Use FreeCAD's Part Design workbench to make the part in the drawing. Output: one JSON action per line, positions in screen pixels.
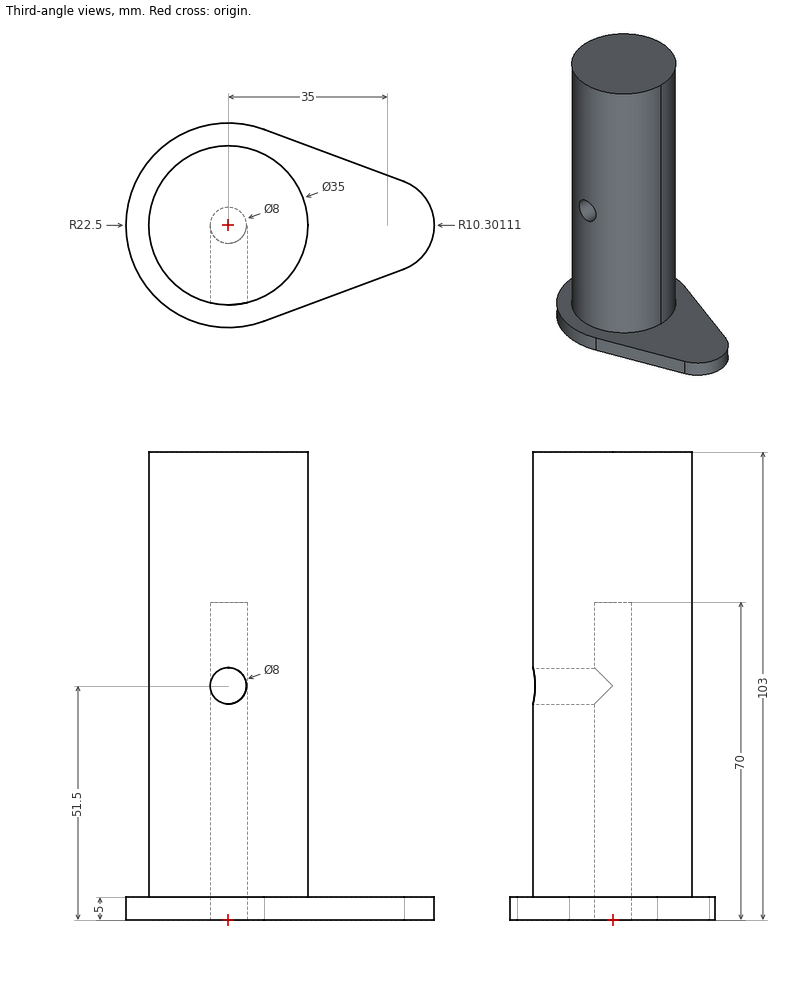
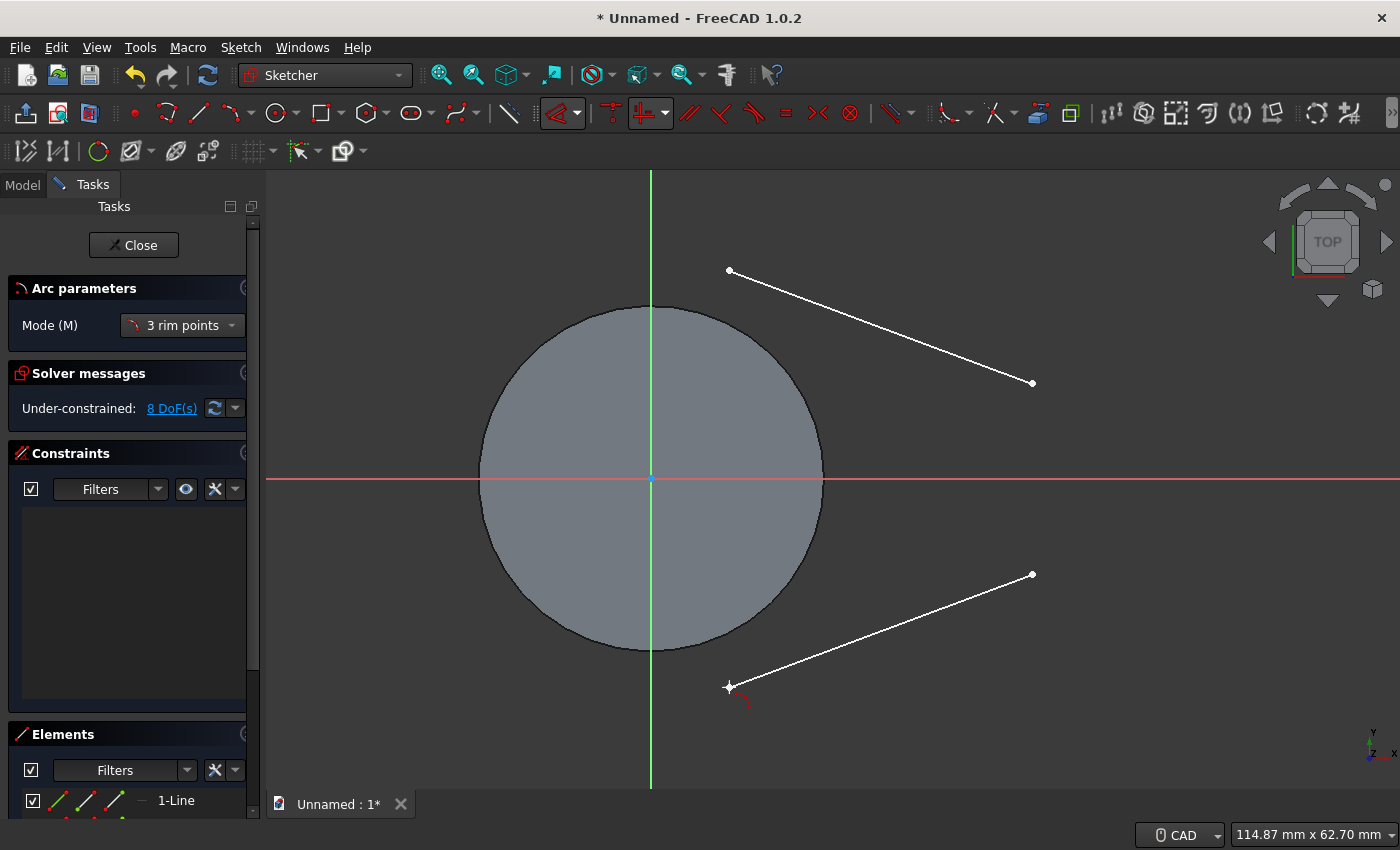
{"action": "left_click", "coordinate": [1032, 384]}
{"action": "left_click", "coordinate": [1032, 575]}
{"action": "left_click", "coordinate": [1096, 503]}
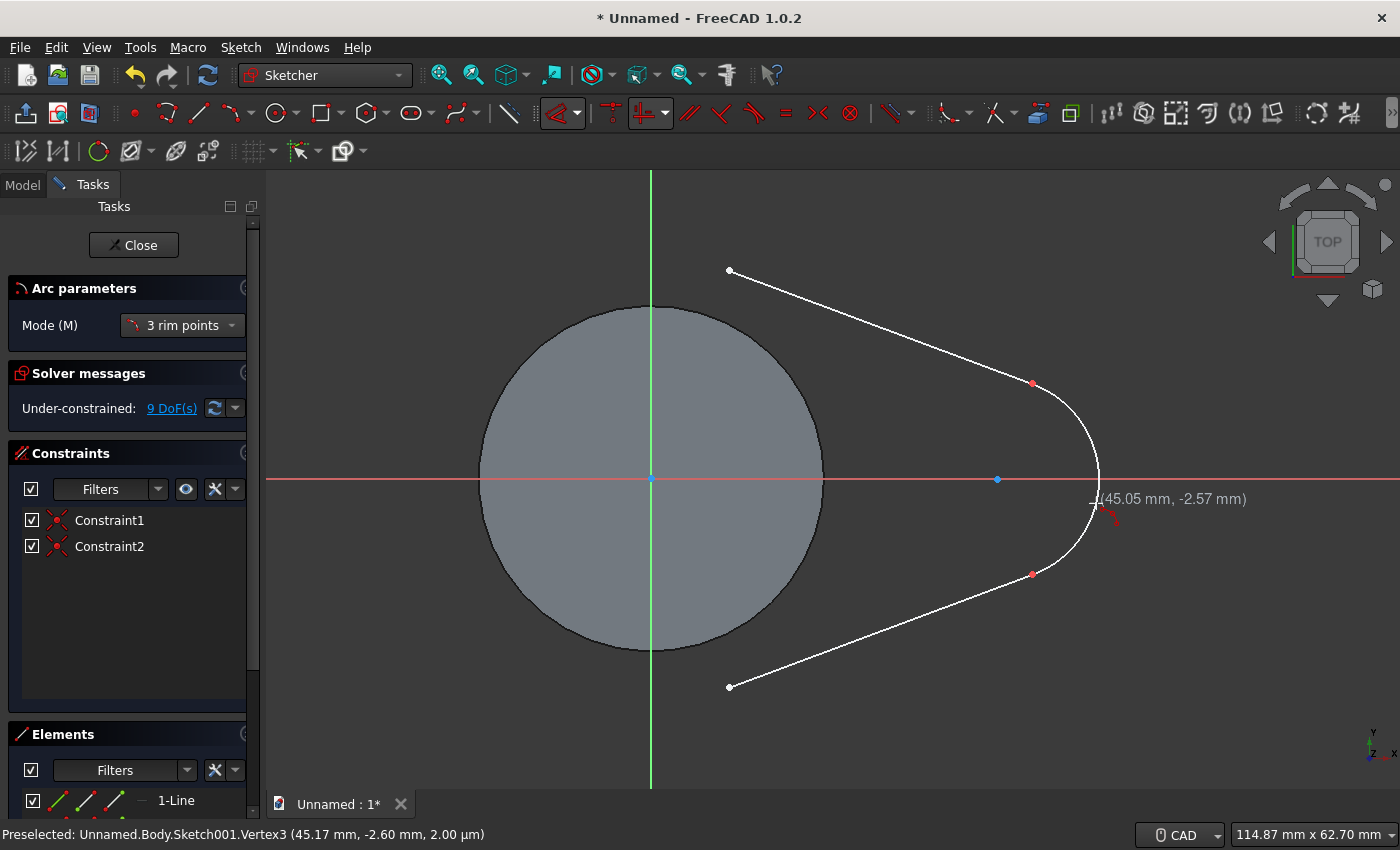
{"action": "left_click", "coordinate": [729, 688]}
{"action": "left_click", "coordinate": [729, 271]}
{"action": "left_click", "coordinate": [445, 395]}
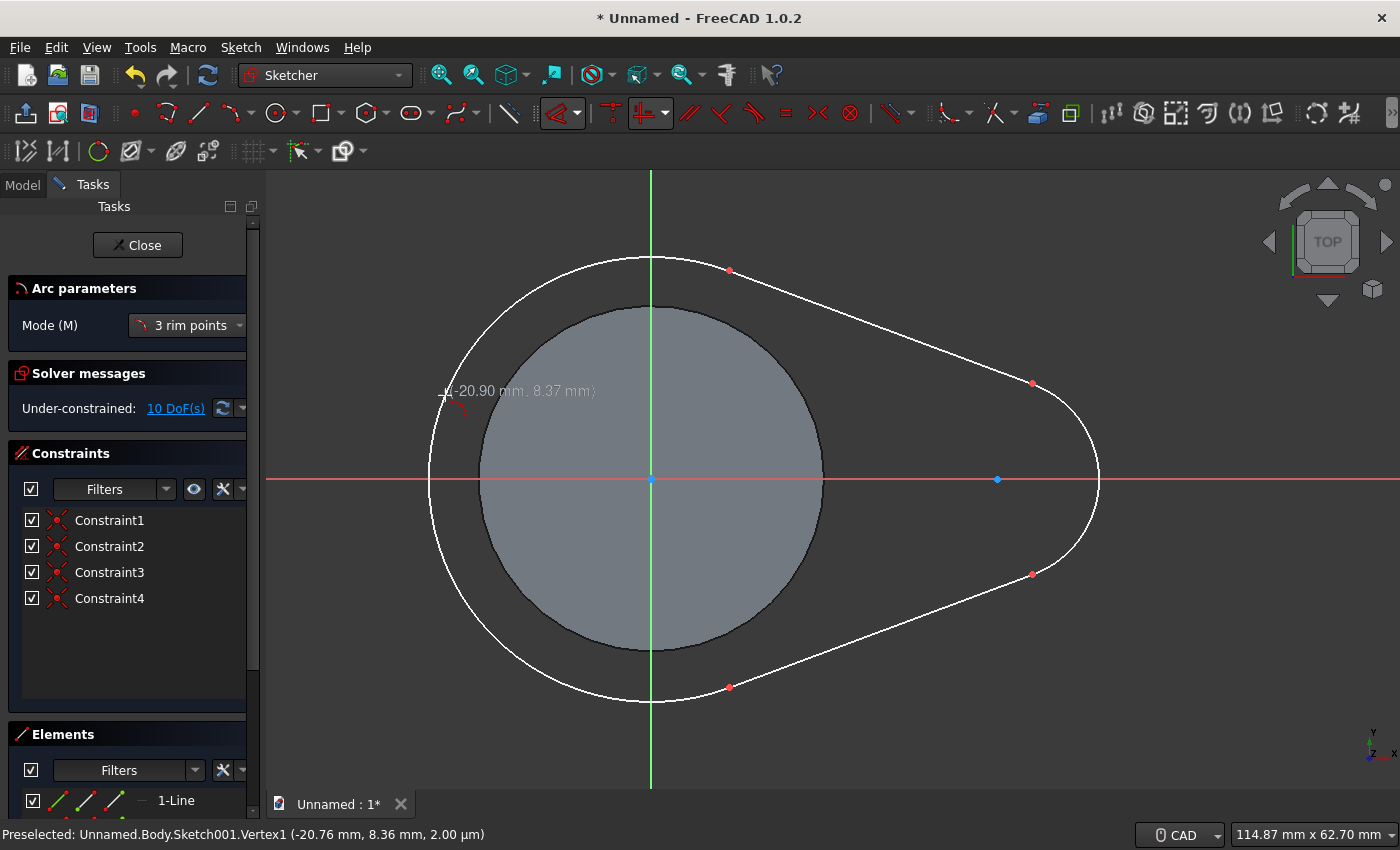
{"action": "left_click", "coordinate": [276, 114]}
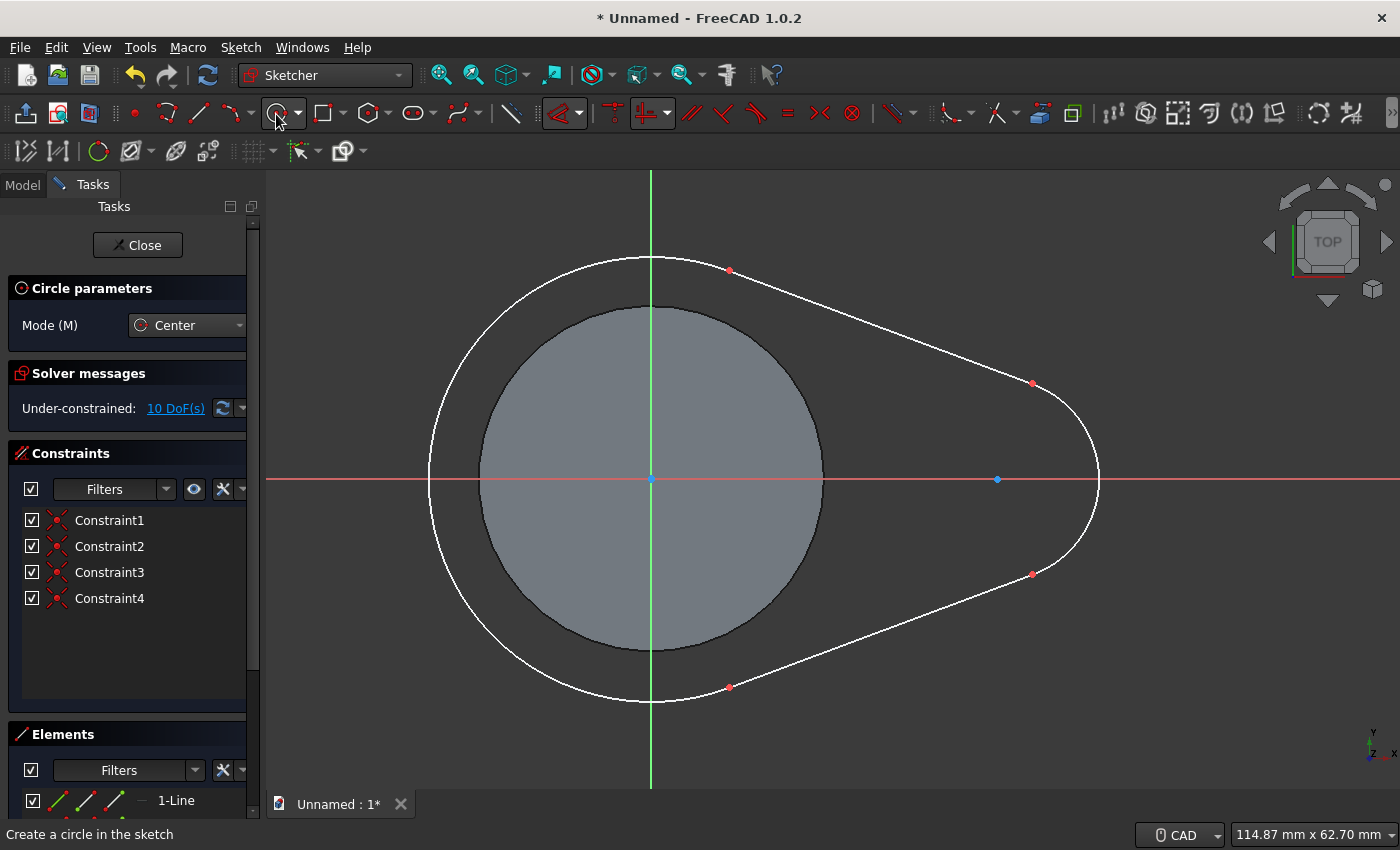
{"action": "left_click", "coordinate": [651, 479]}
{"action": "left_click", "coordinate": [773, 357]}
{"action": "key", "text": "Escape"}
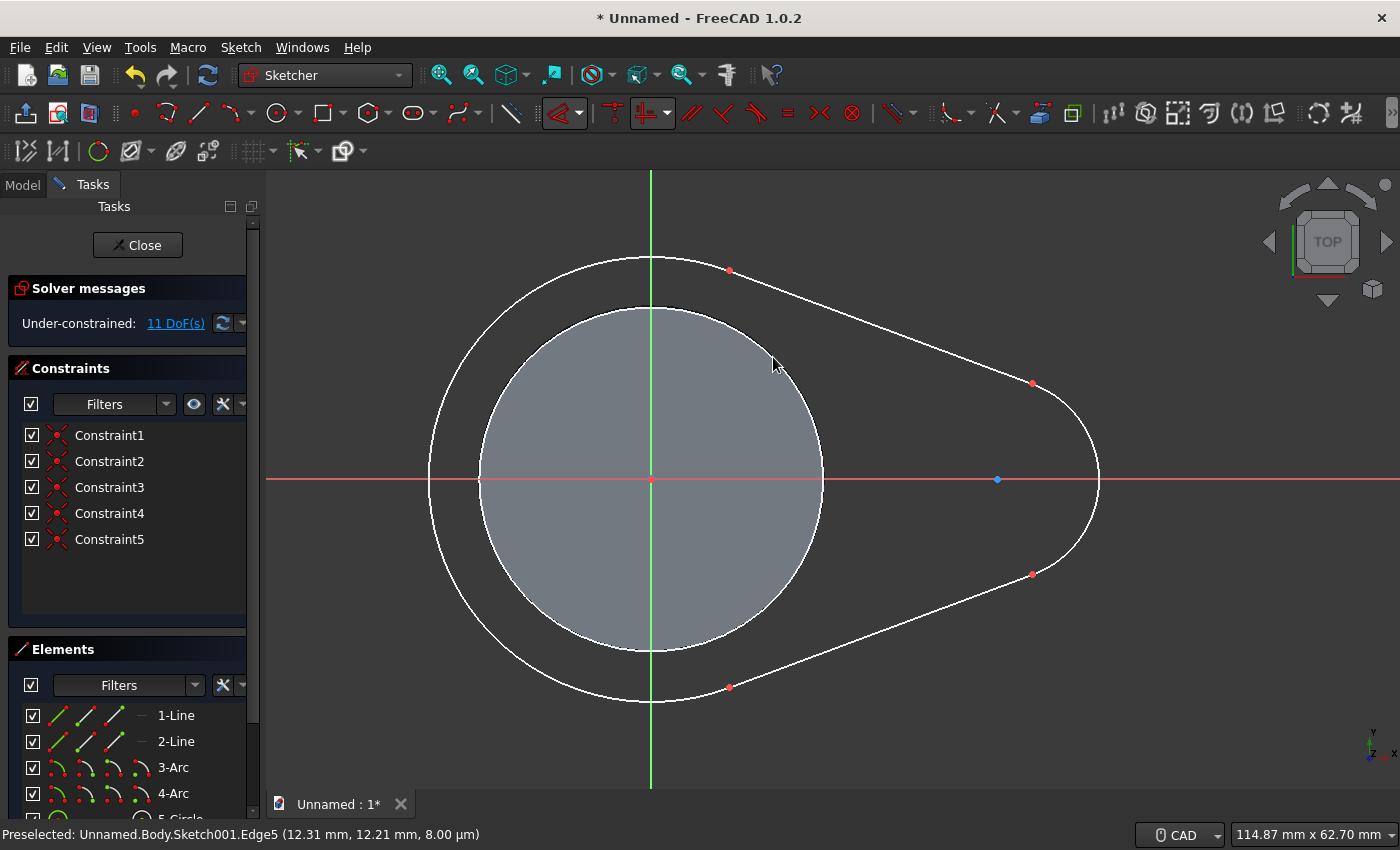
{"action": "left_click", "coordinate": [820, 305]}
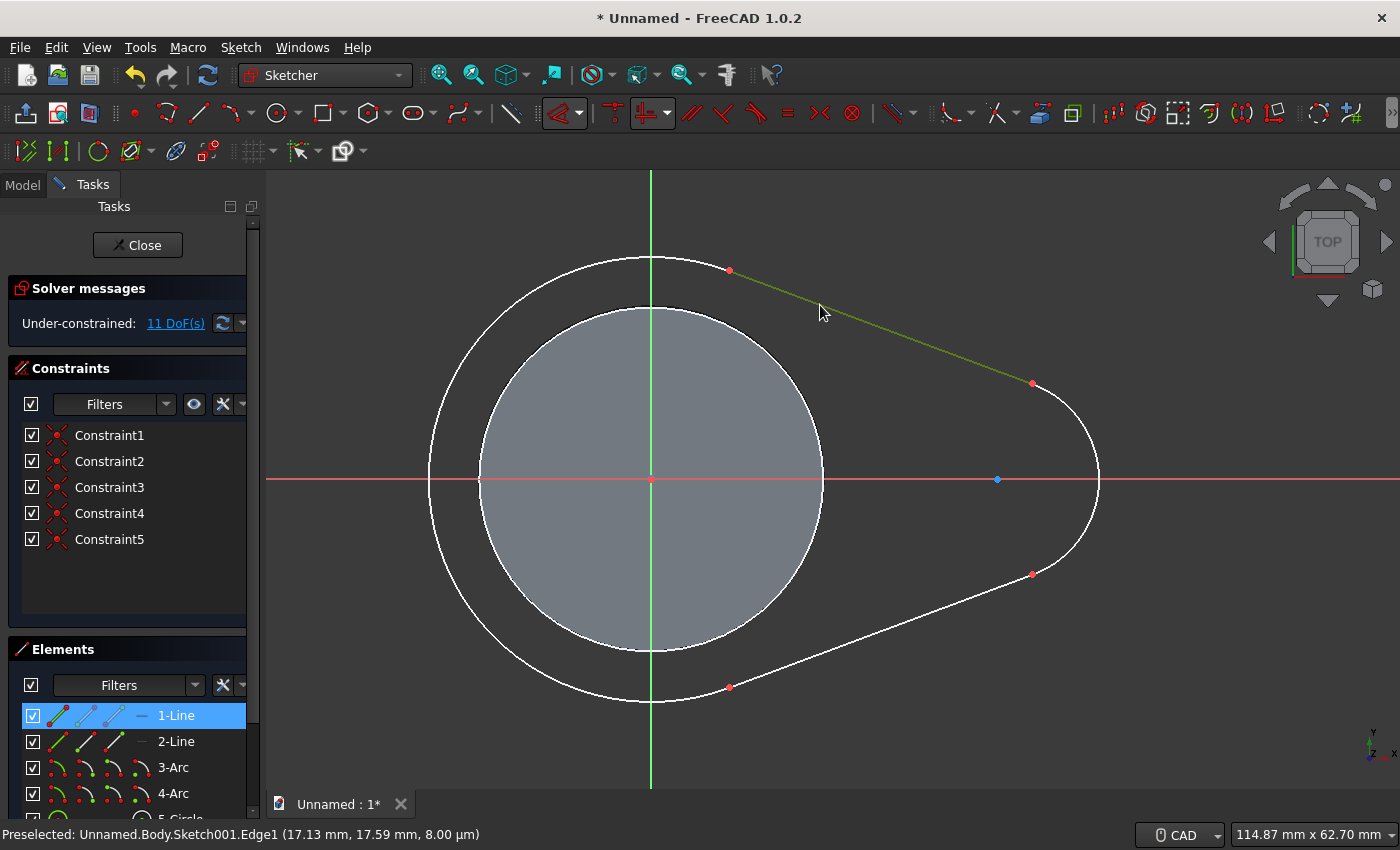
{"action": "left_click", "coordinate": [1087, 527]}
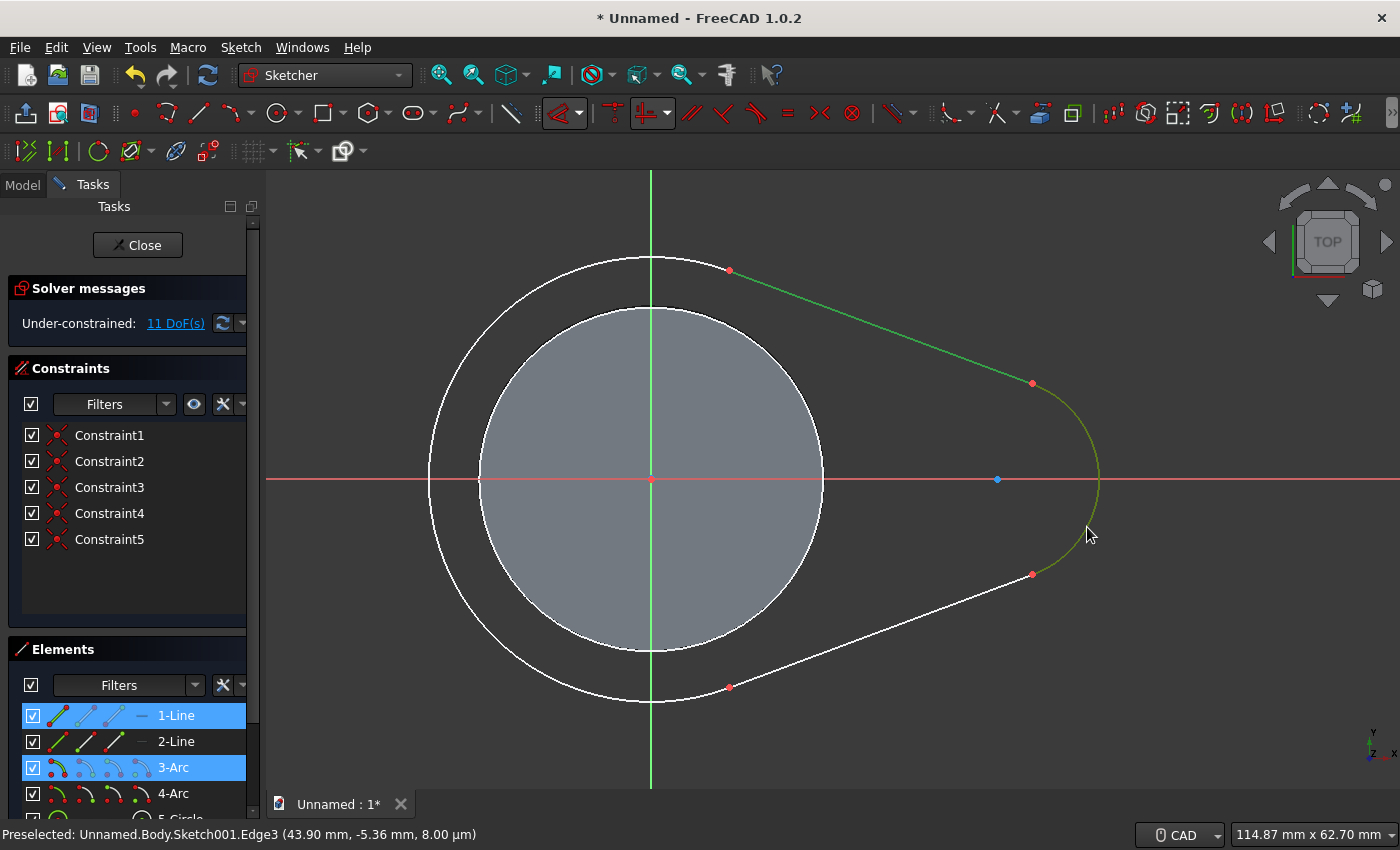
{"action": "left_click", "coordinate": [756, 114]}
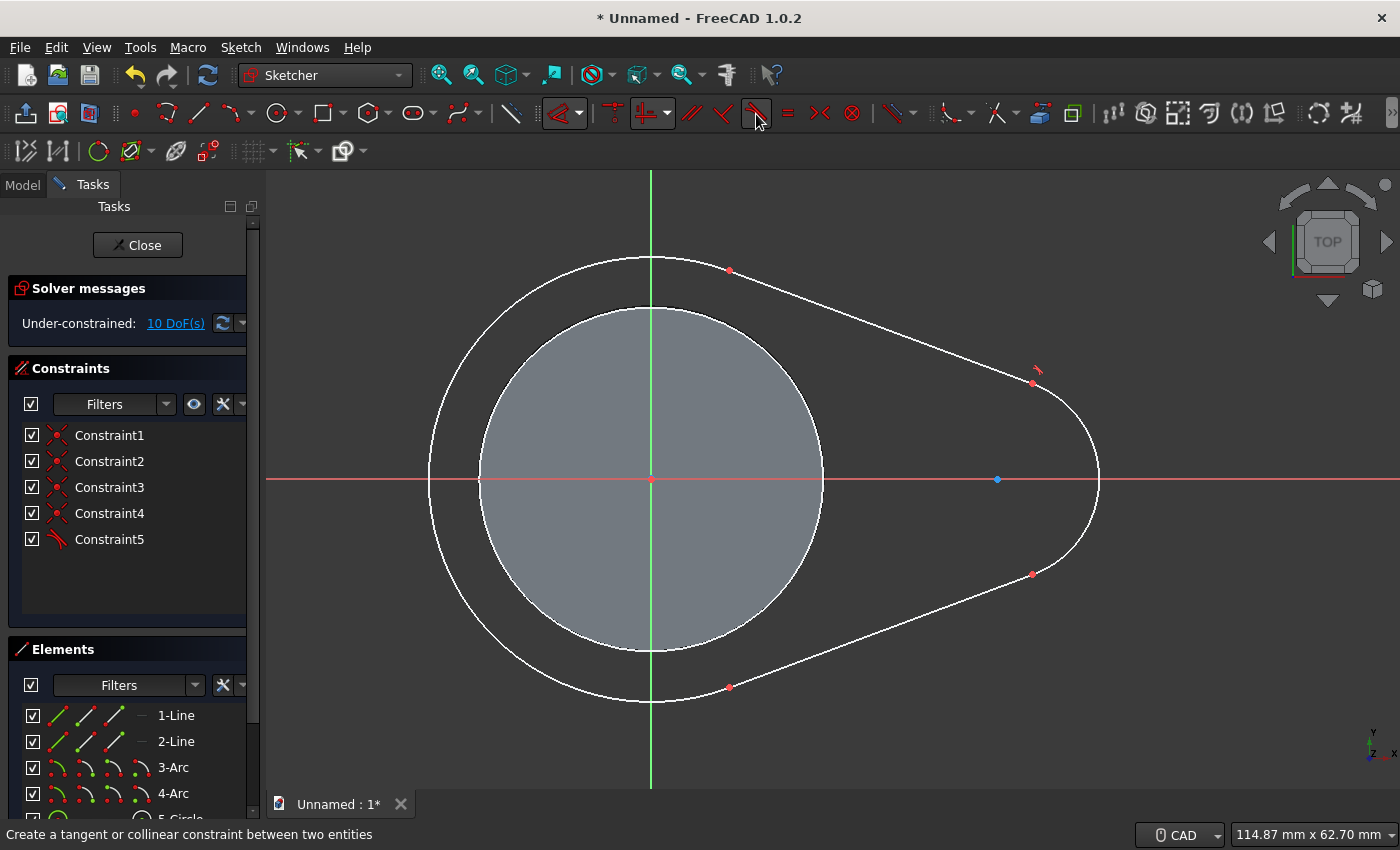
{"action": "left_click", "coordinate": [820, 305]}